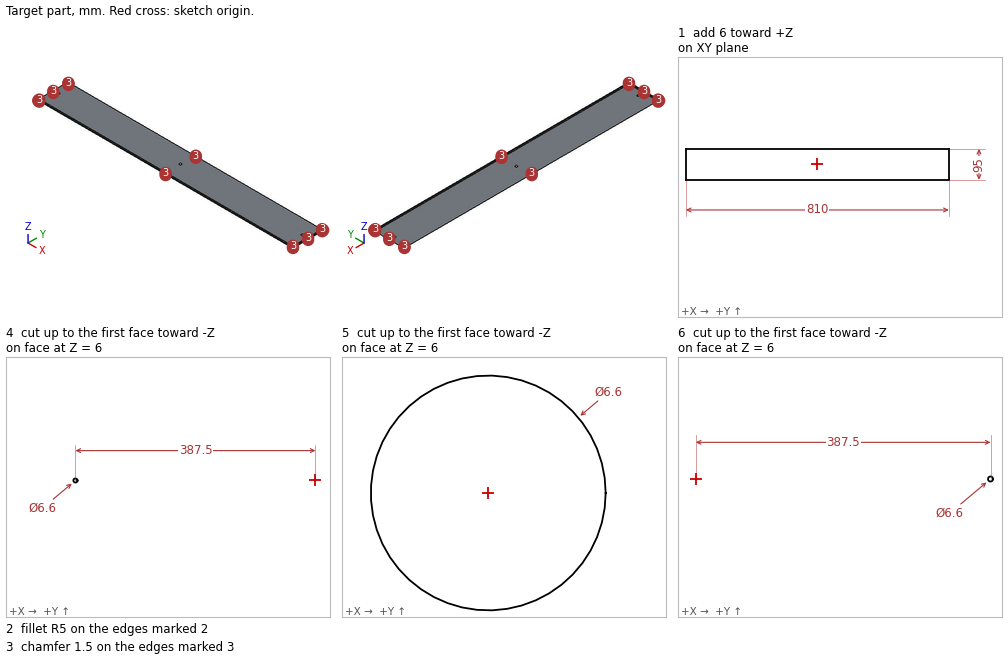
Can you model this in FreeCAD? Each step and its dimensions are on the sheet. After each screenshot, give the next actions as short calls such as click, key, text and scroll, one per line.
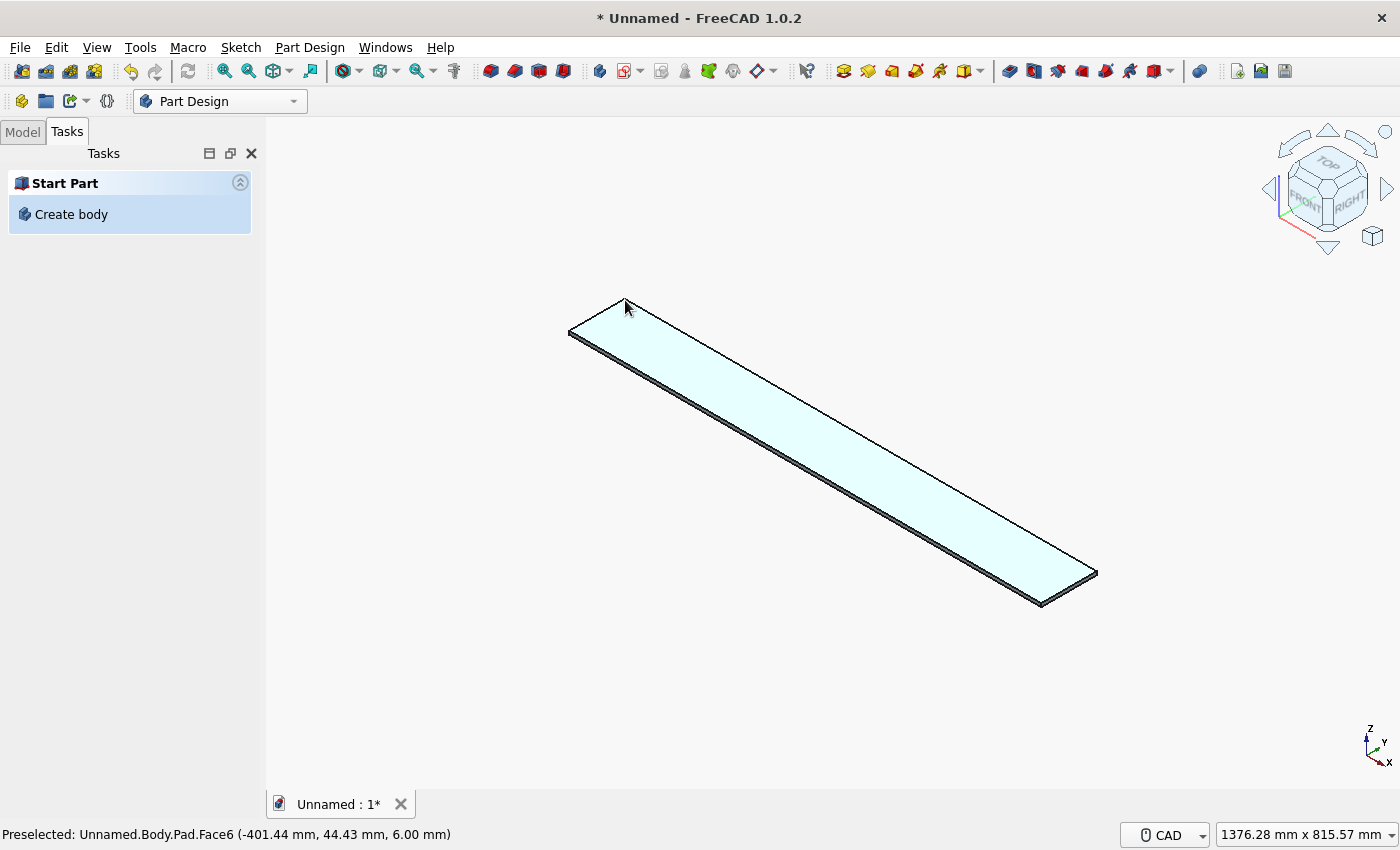
key(2)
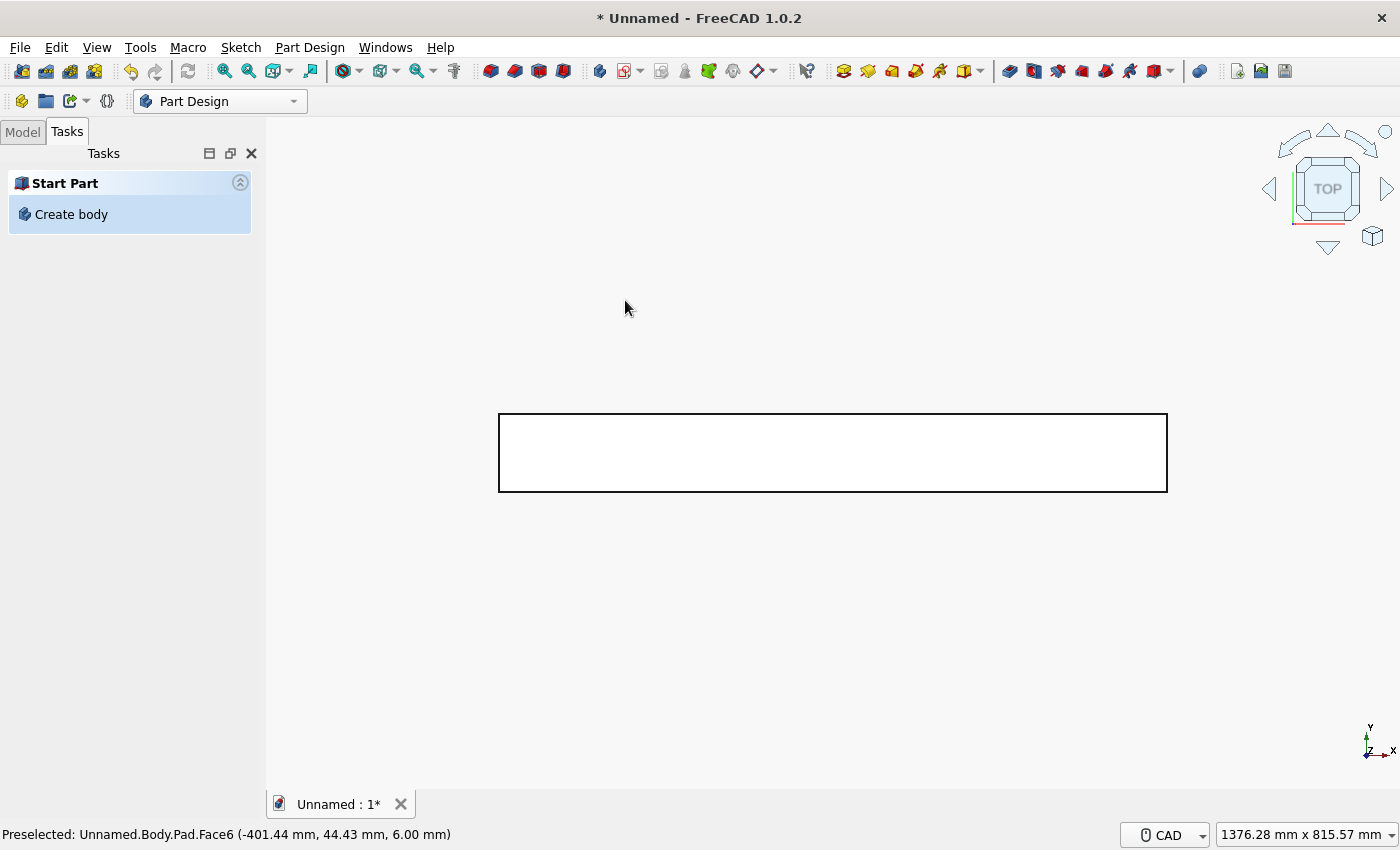
scroll(499, 413, up, 11)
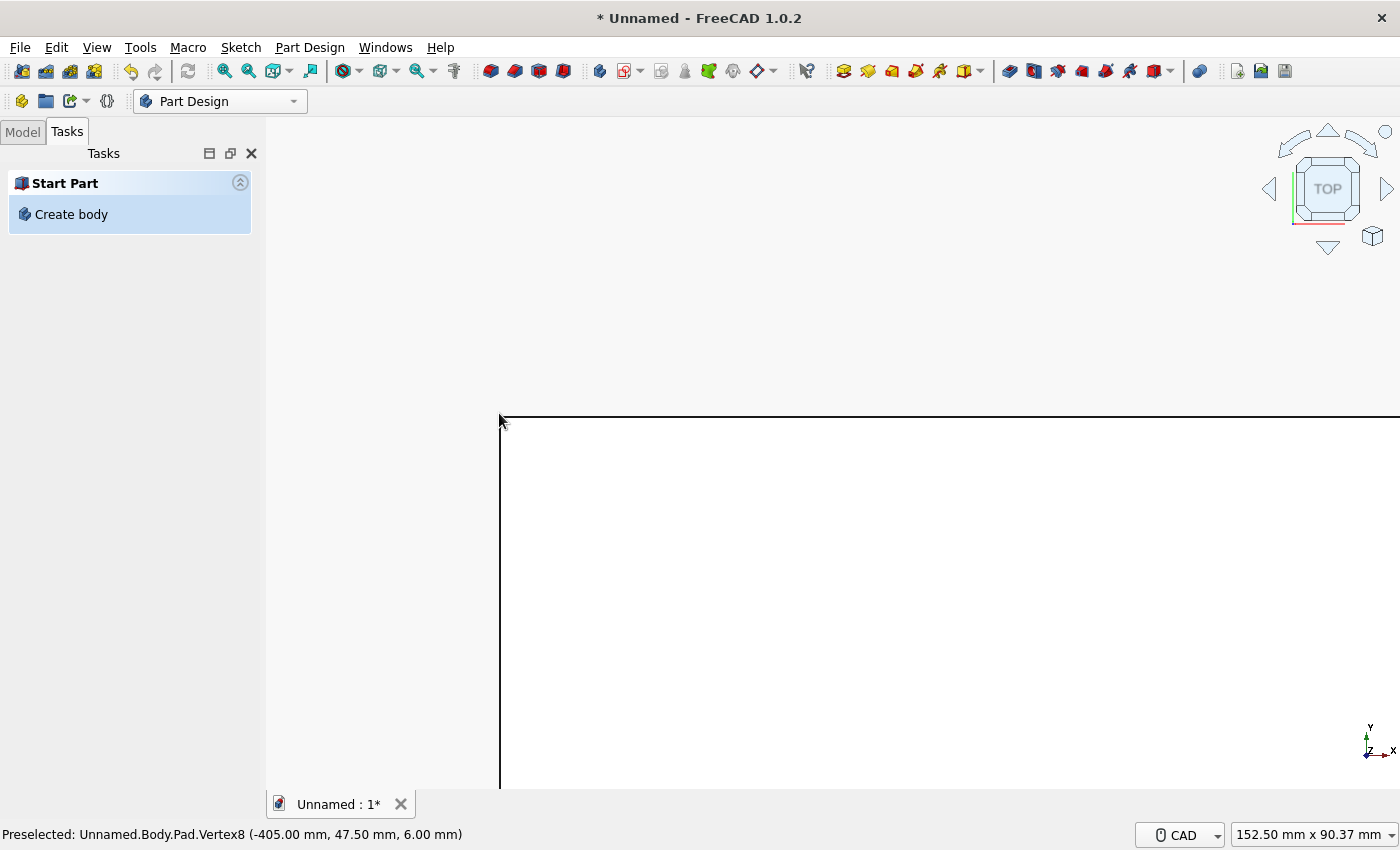
key(v)
key(f)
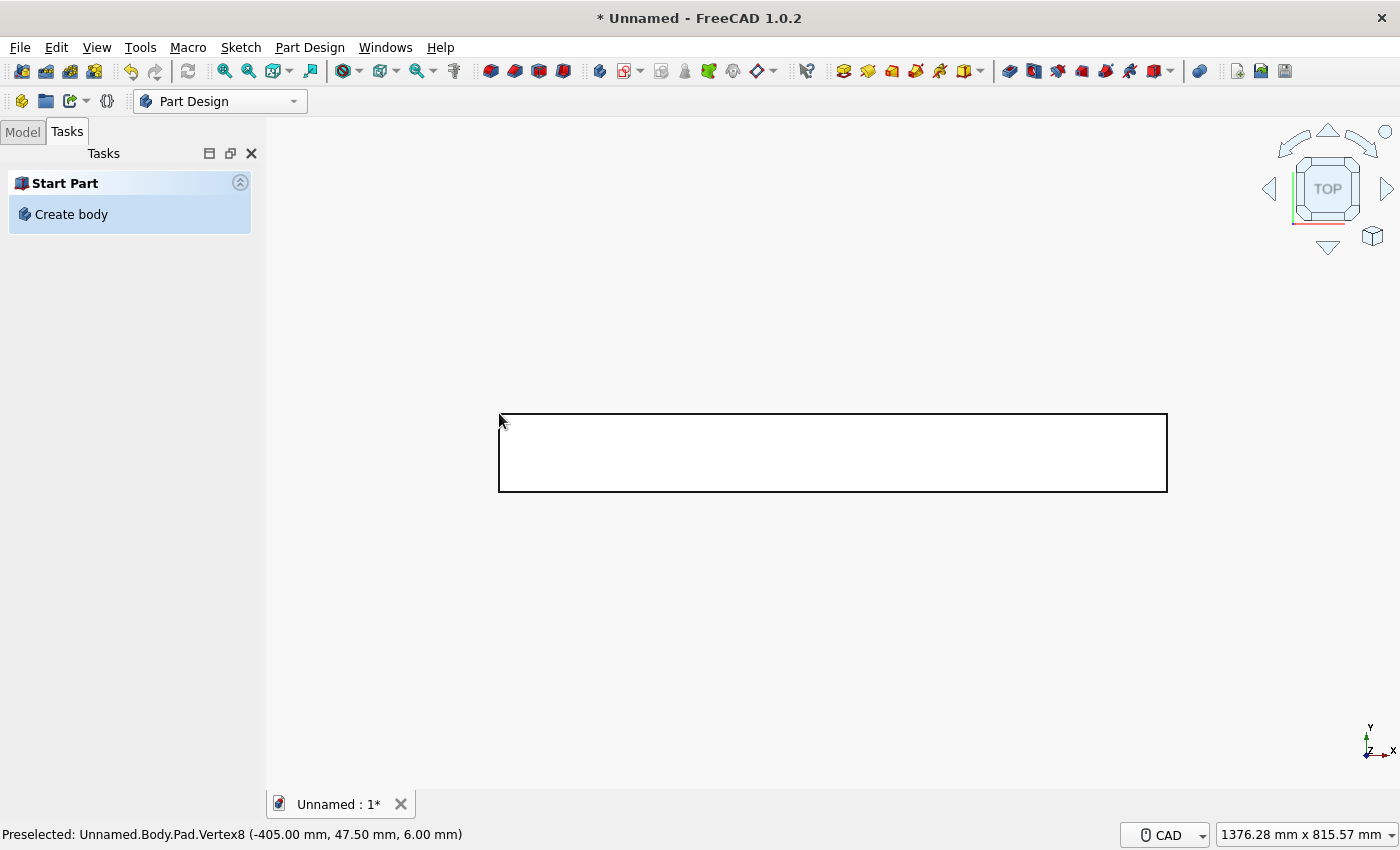
key(1)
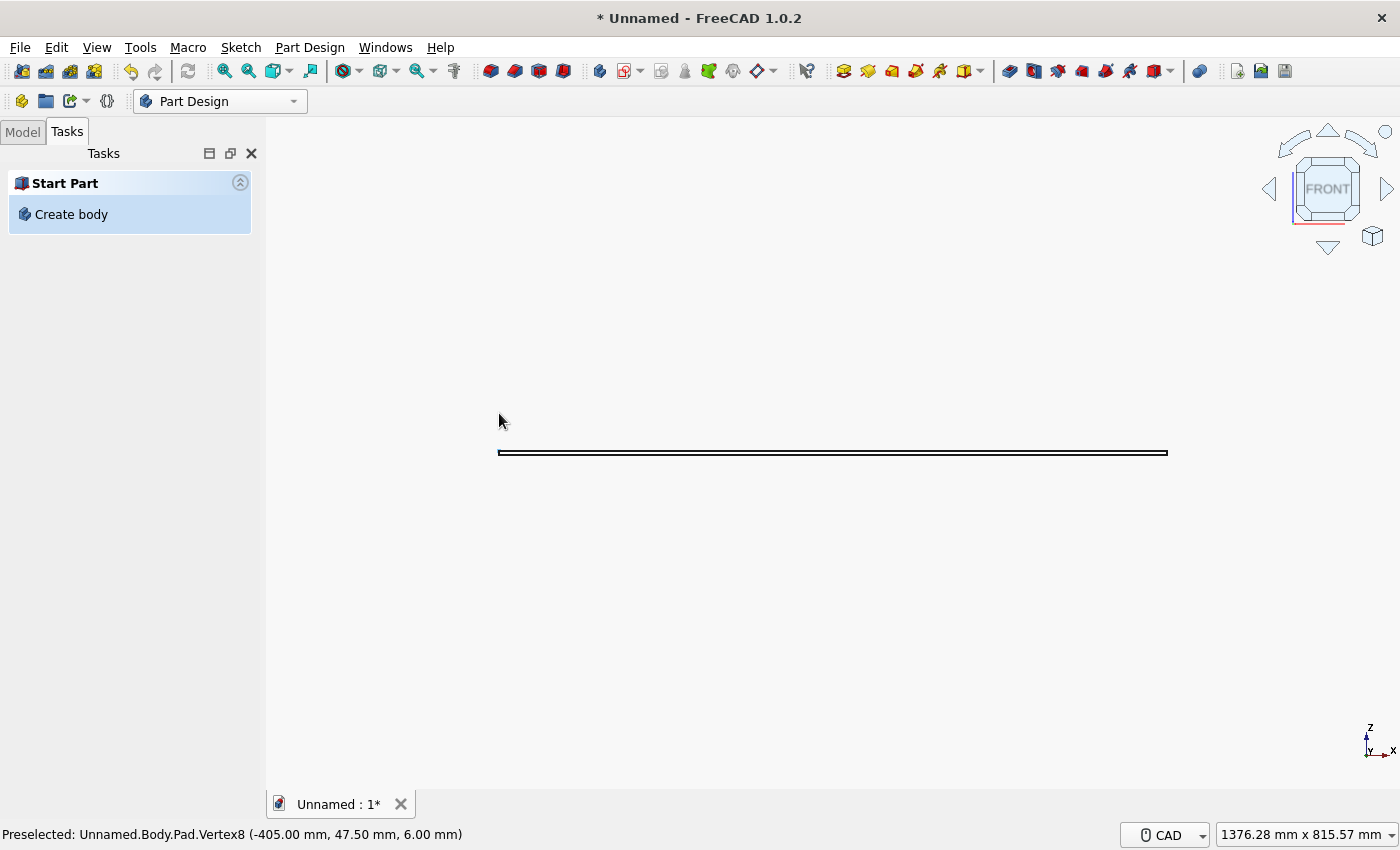
scroll(499, 452, up, 11)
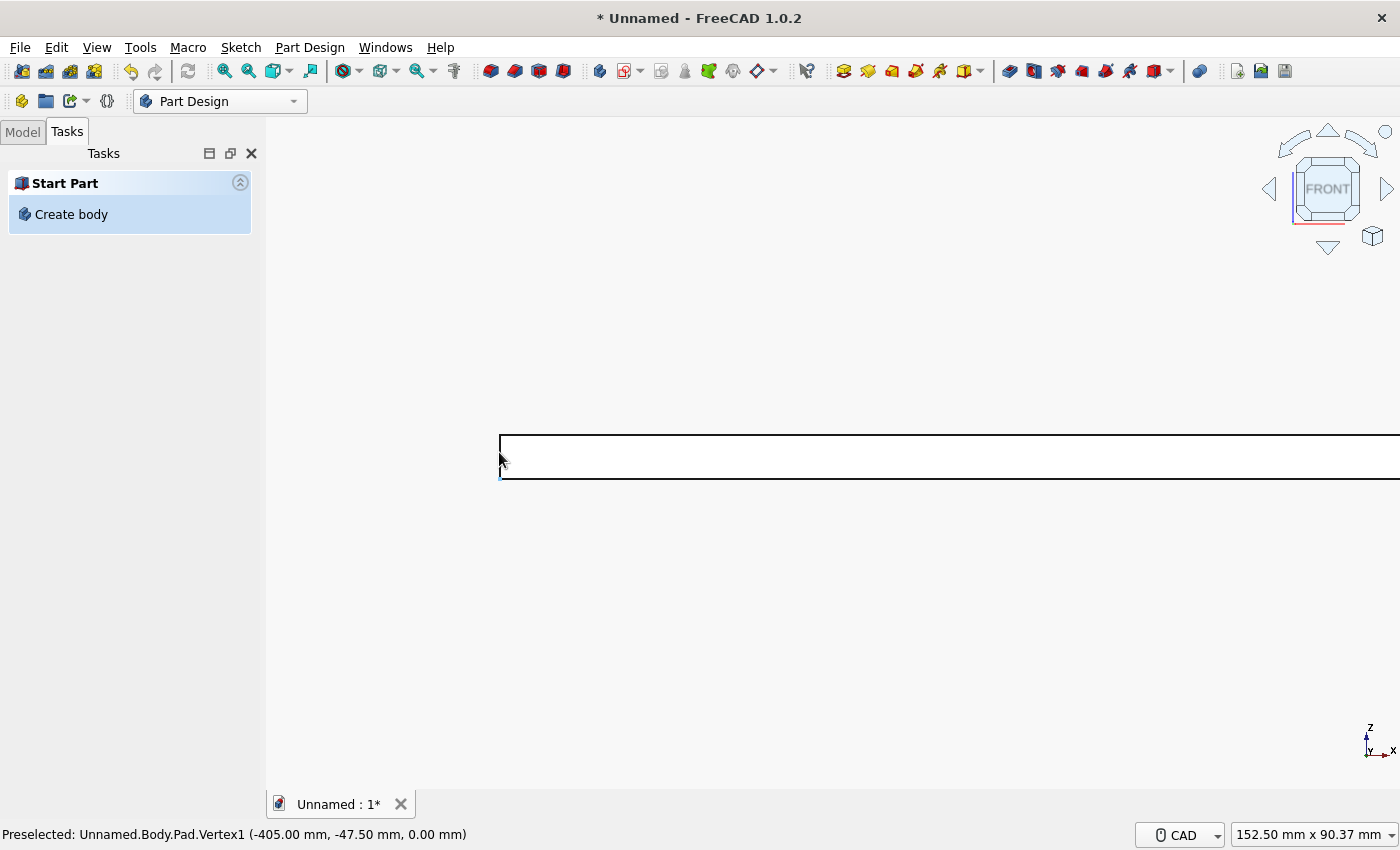
click(500, 456)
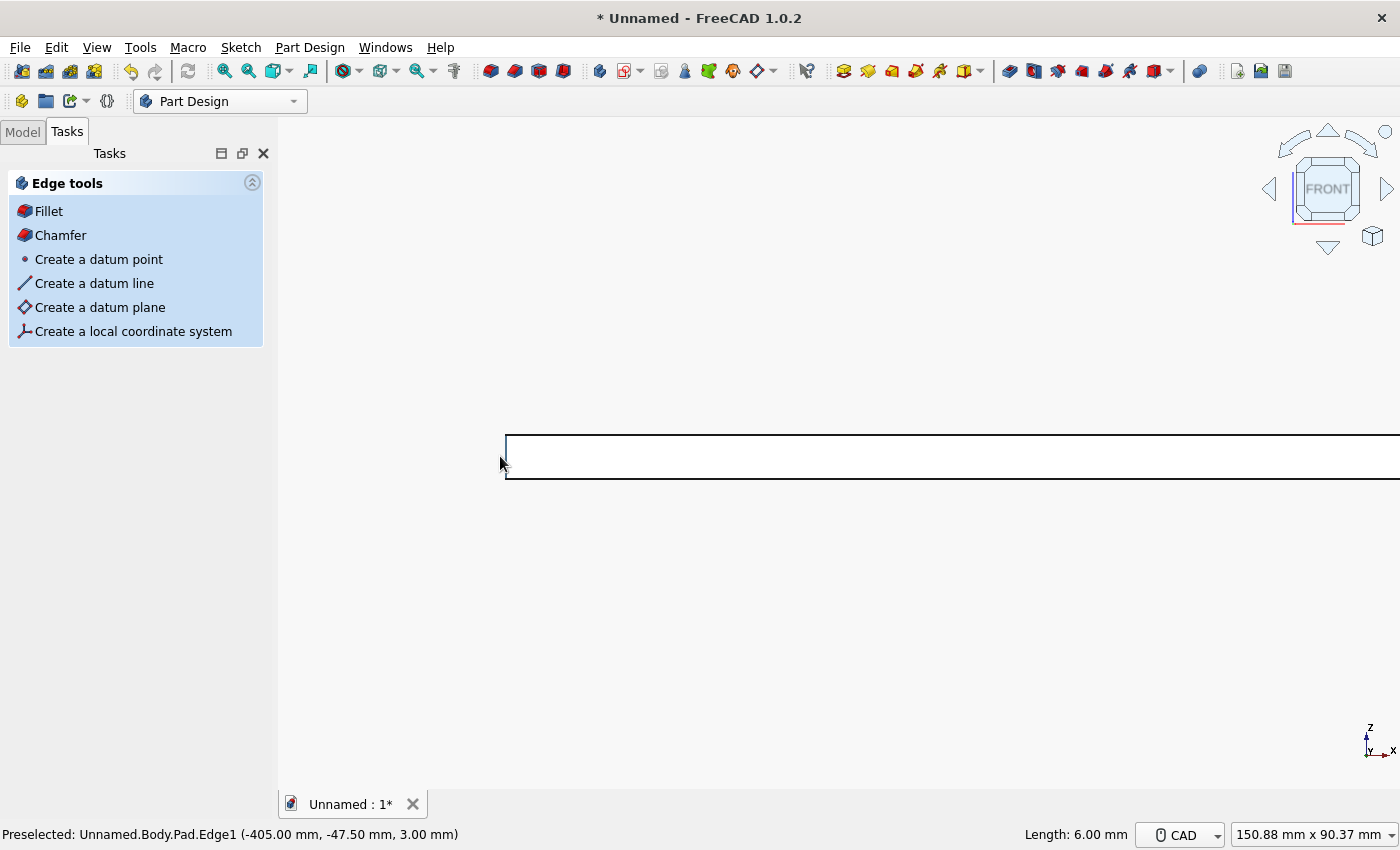
key(v)
key(f)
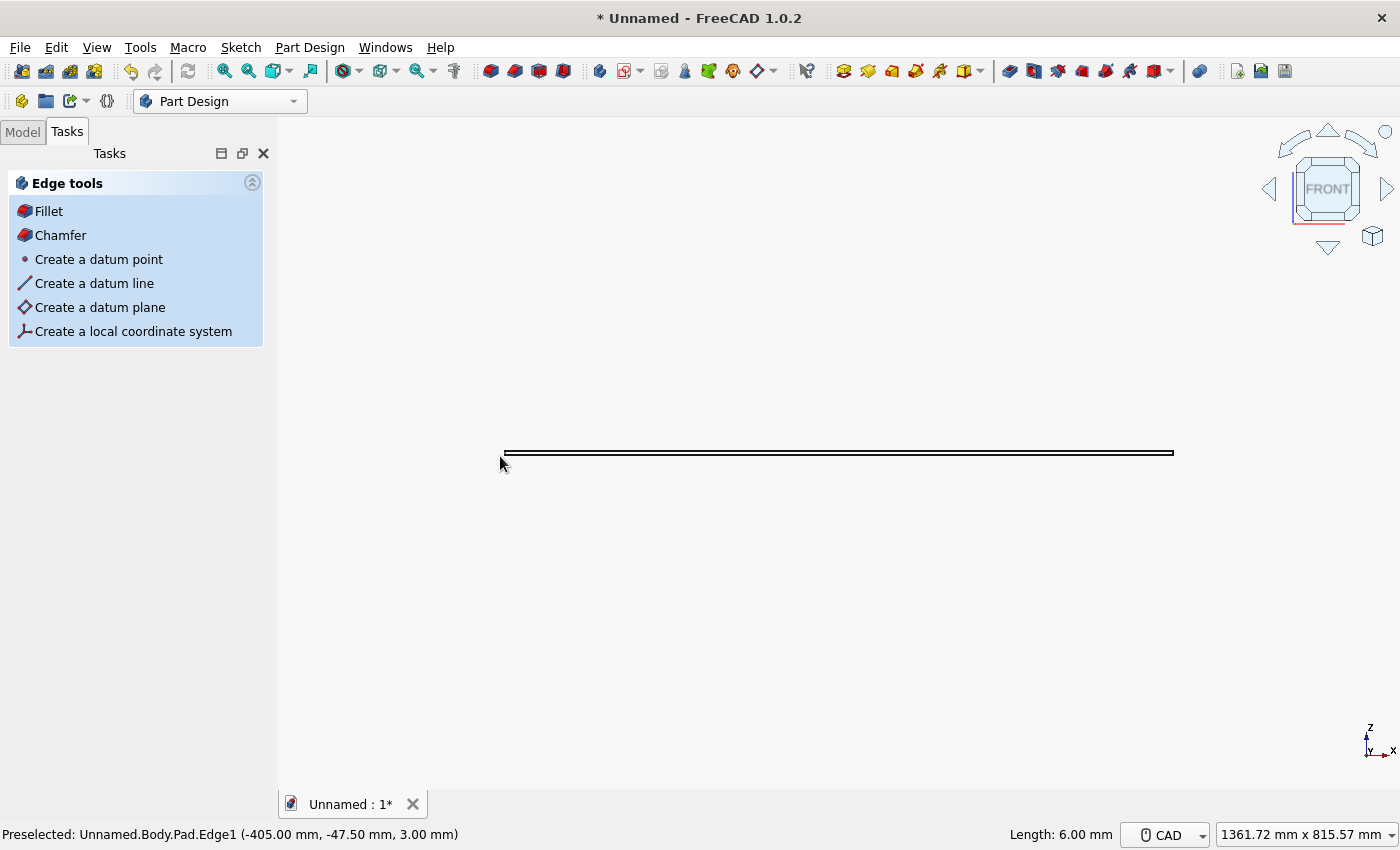
key(3)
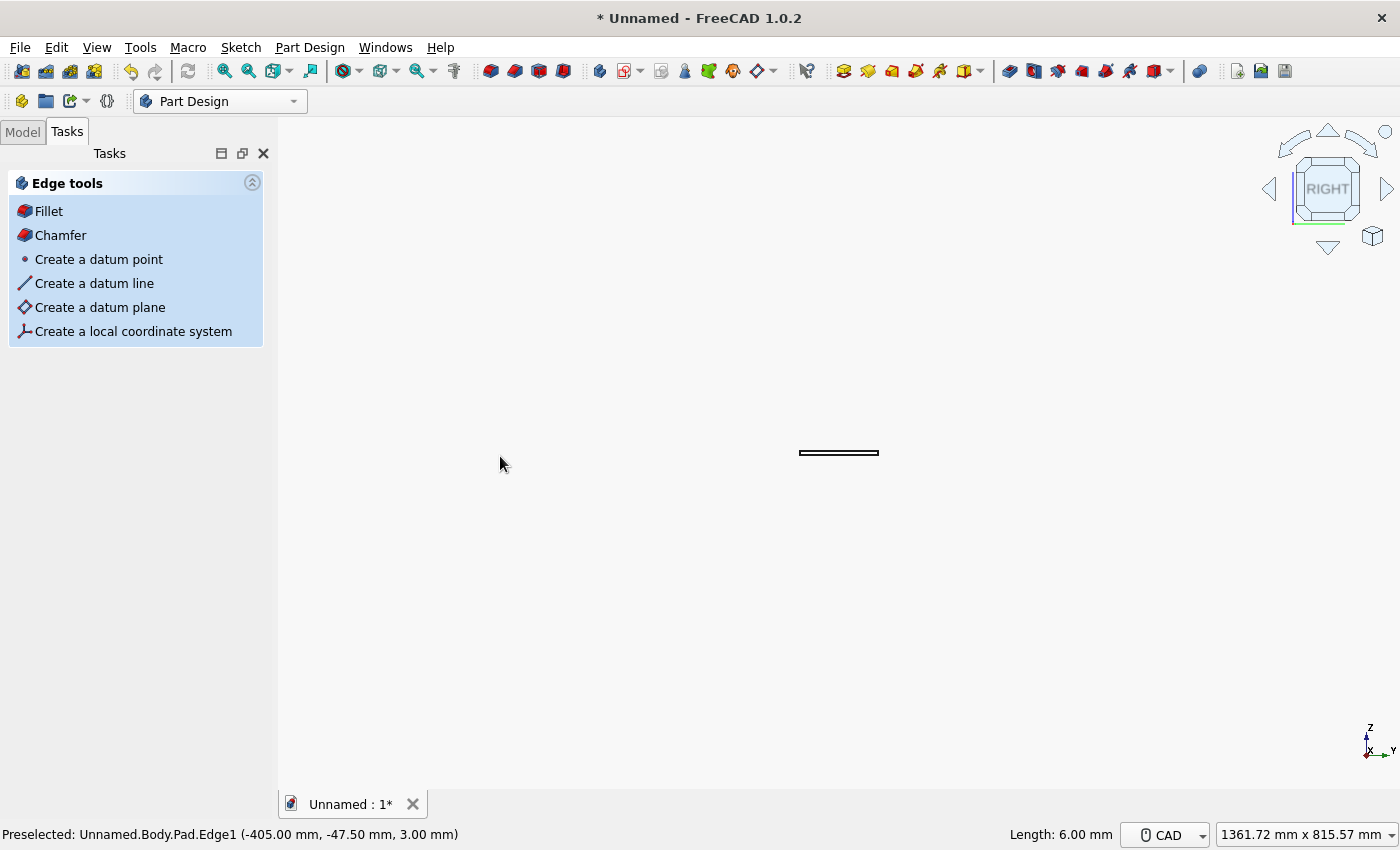
key(v)
key(f)